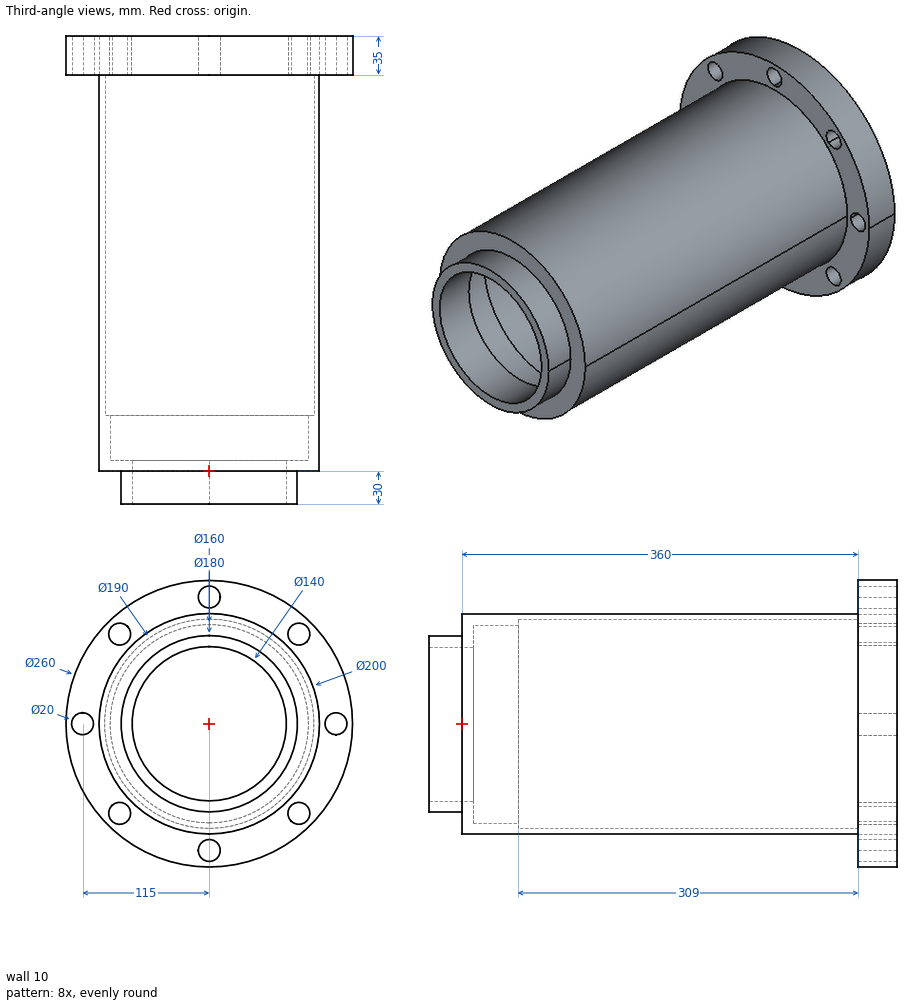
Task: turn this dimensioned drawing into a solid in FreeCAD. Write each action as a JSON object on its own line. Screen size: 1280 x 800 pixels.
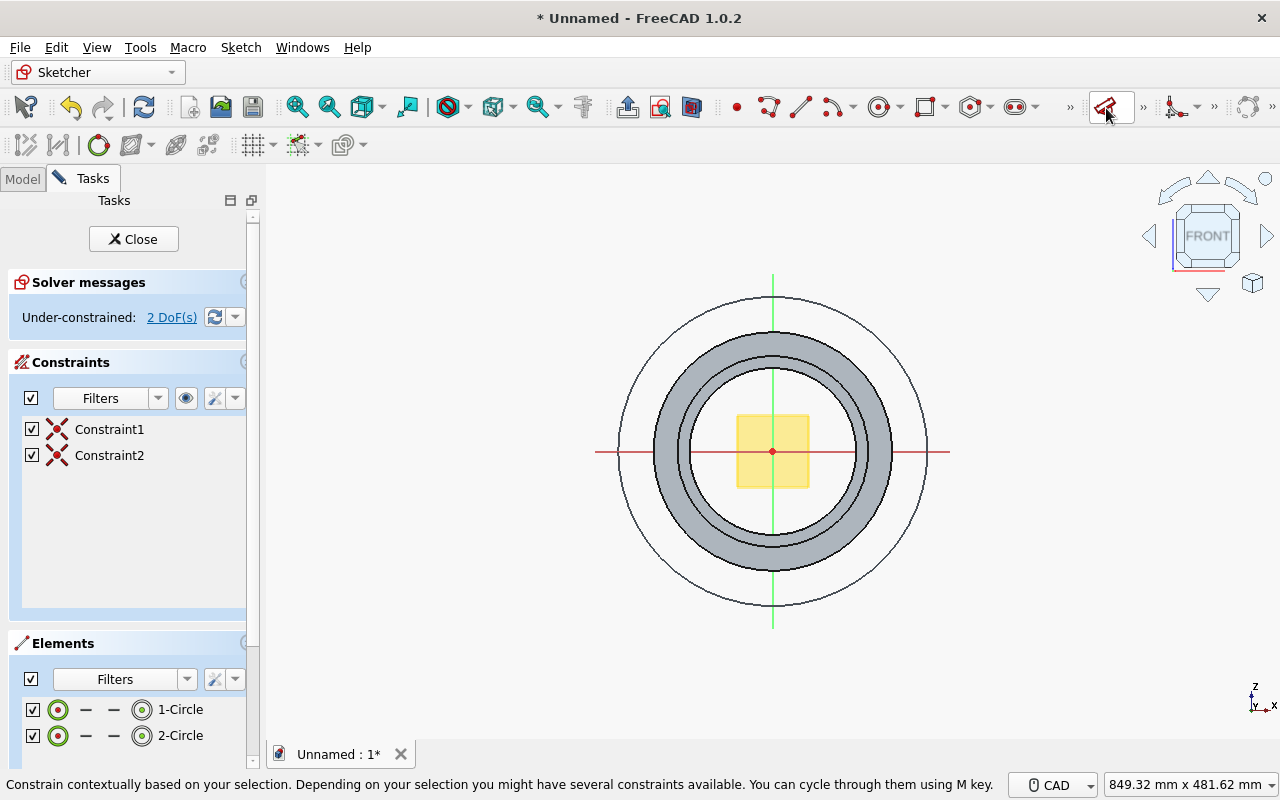
{"action": "left_click", "coordinate": [882, 342]}
{"action": "left_click", "coordinate": [905, 319]}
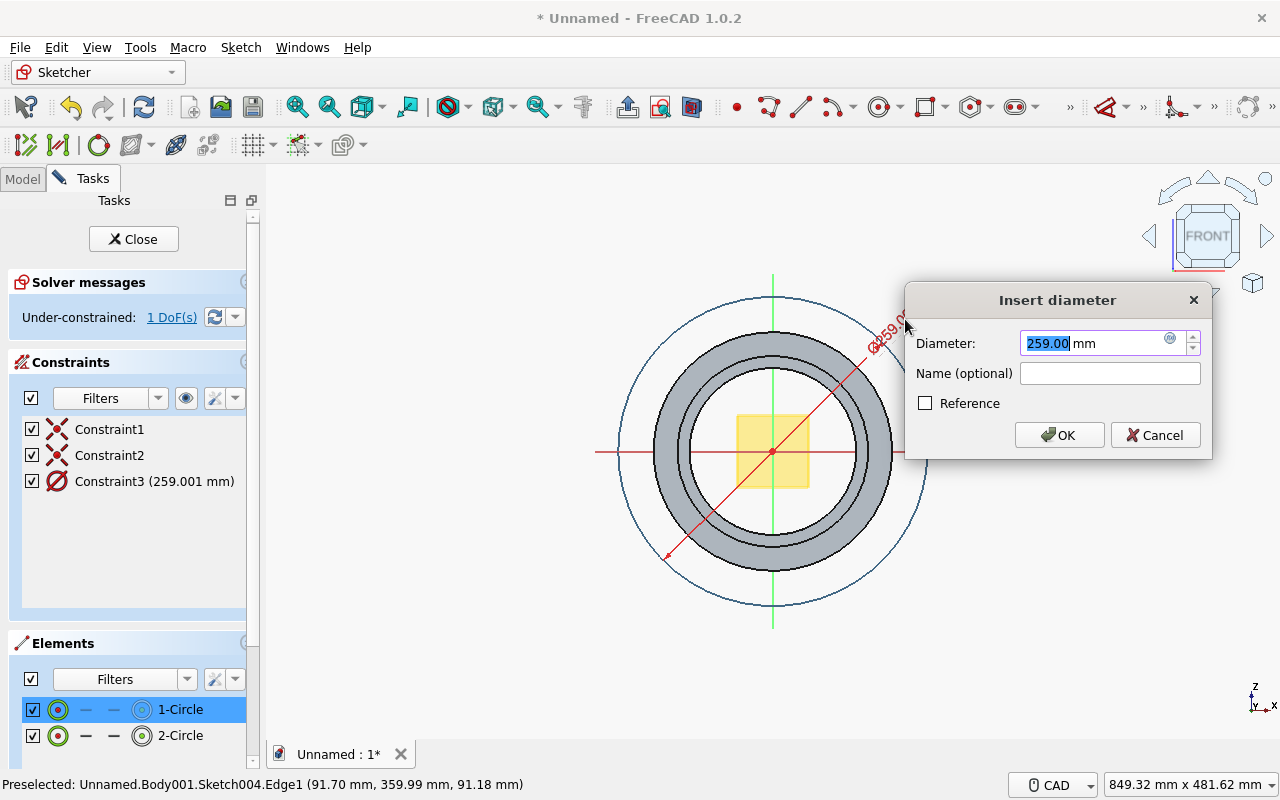
{"action": "type", "text": "260"}
{"action": "key", "text": "Return"}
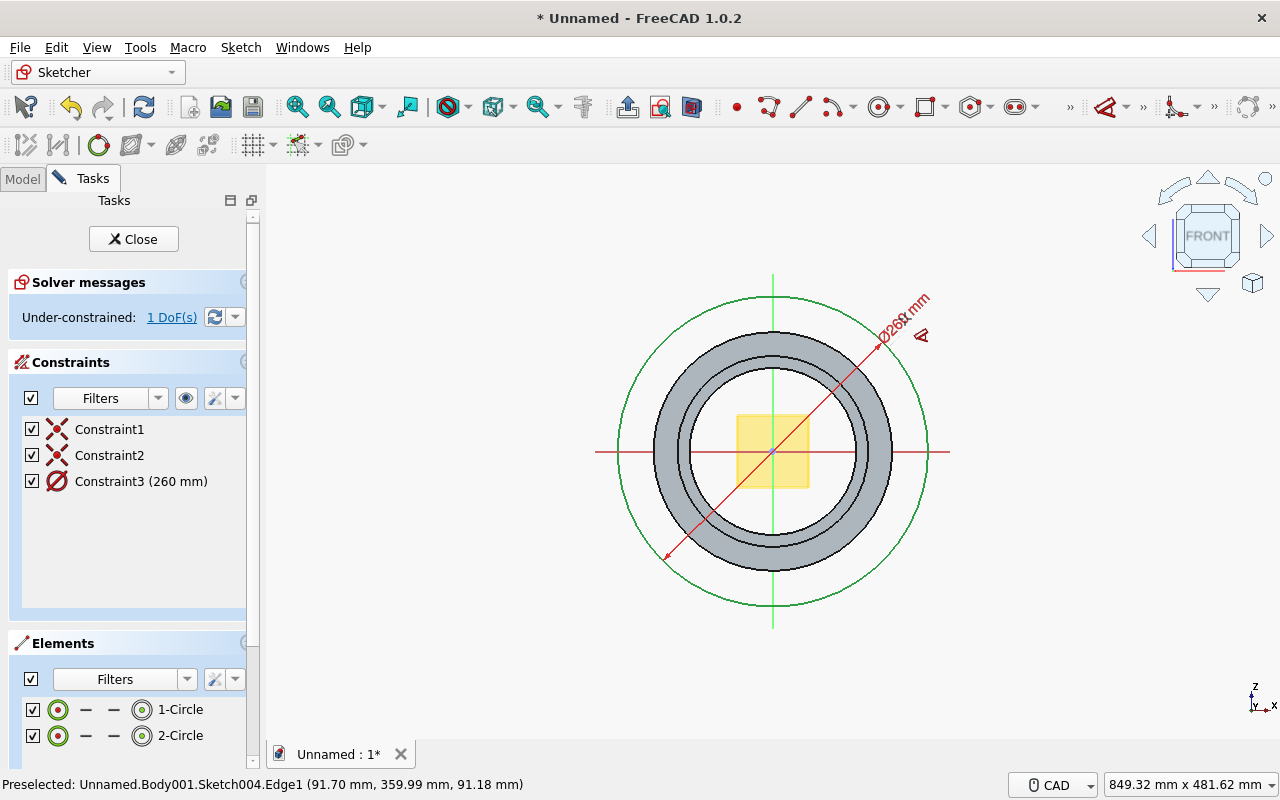
{"action": "left_click", "coordinate": [856, 367]}
{"action": "left_click", "coordinate": [939, 401]}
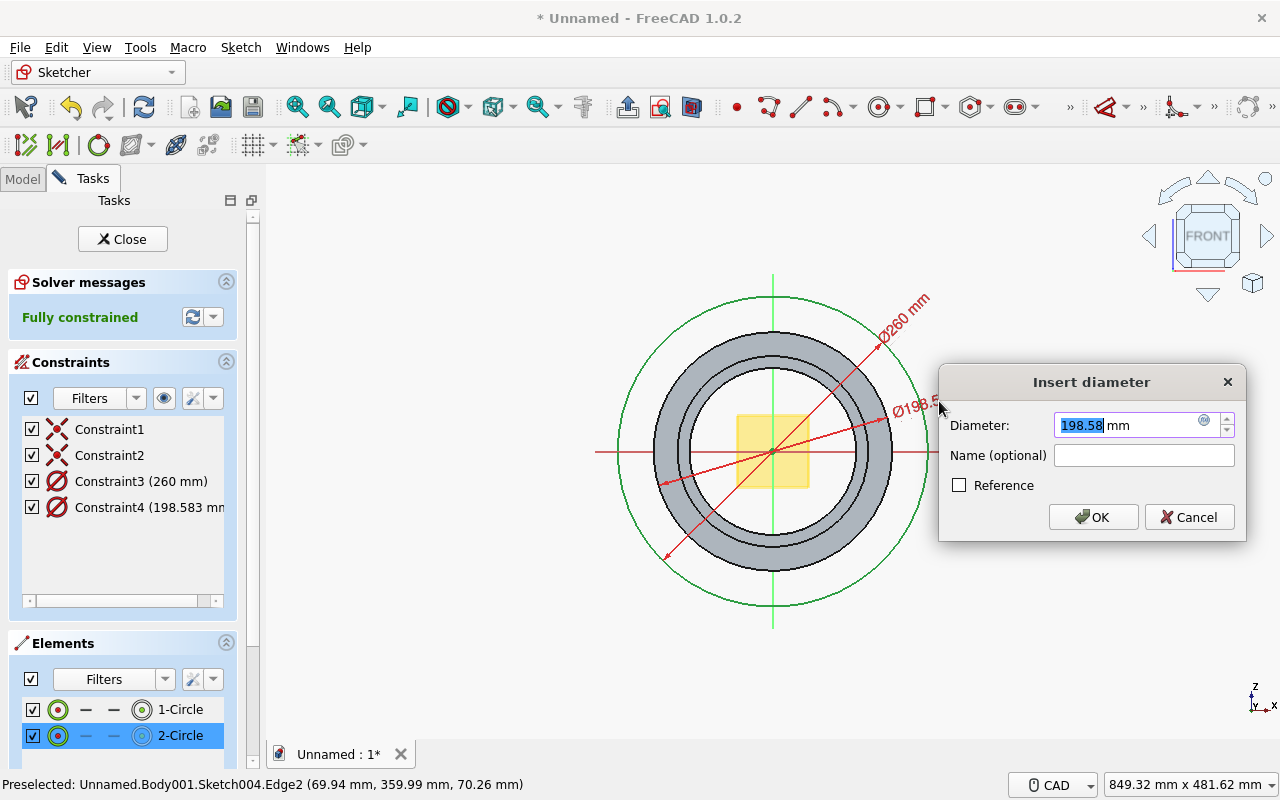
{"action": "type", "text": "200"}
{"action": "key", "text": "Return"}
{"action": "key", "text": "Escape"}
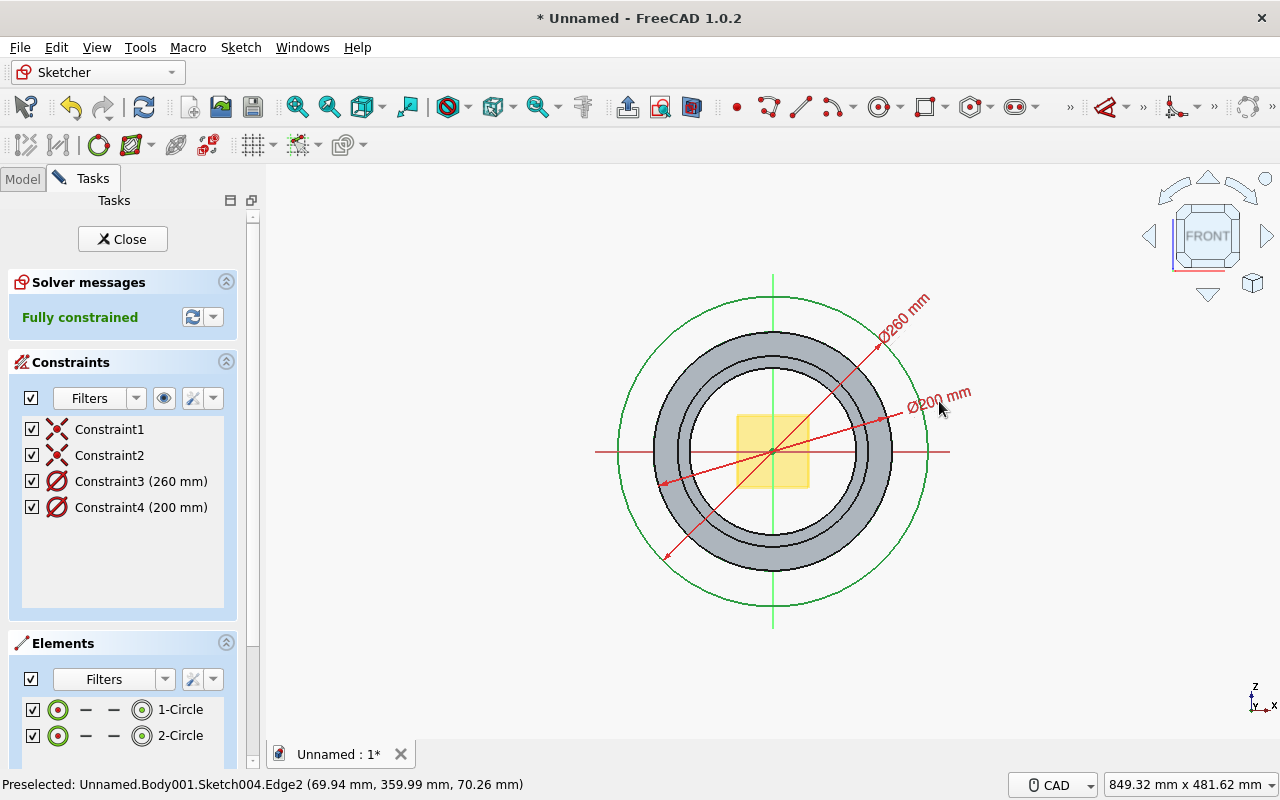
{"action": "left_click", "coordinate": [123, 239]}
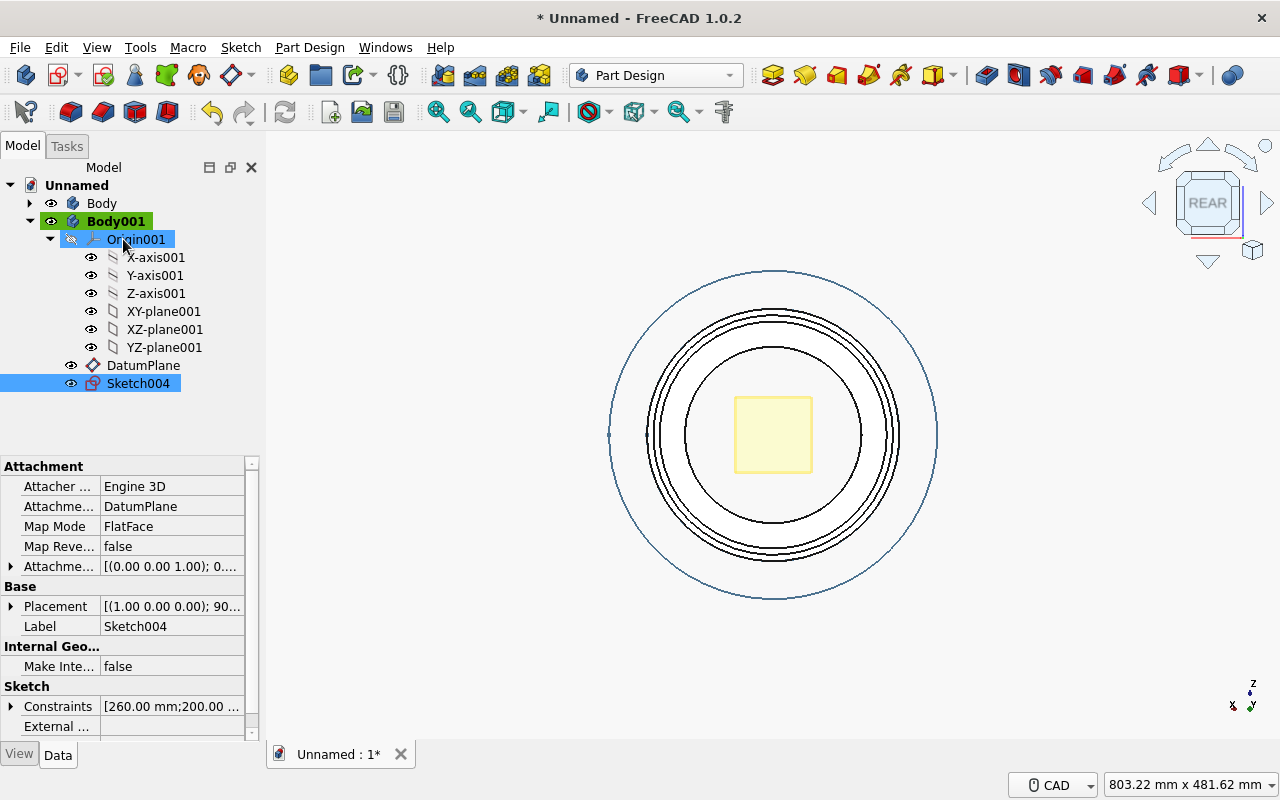
{"action": "left_click", "coordinate": [774, 76]}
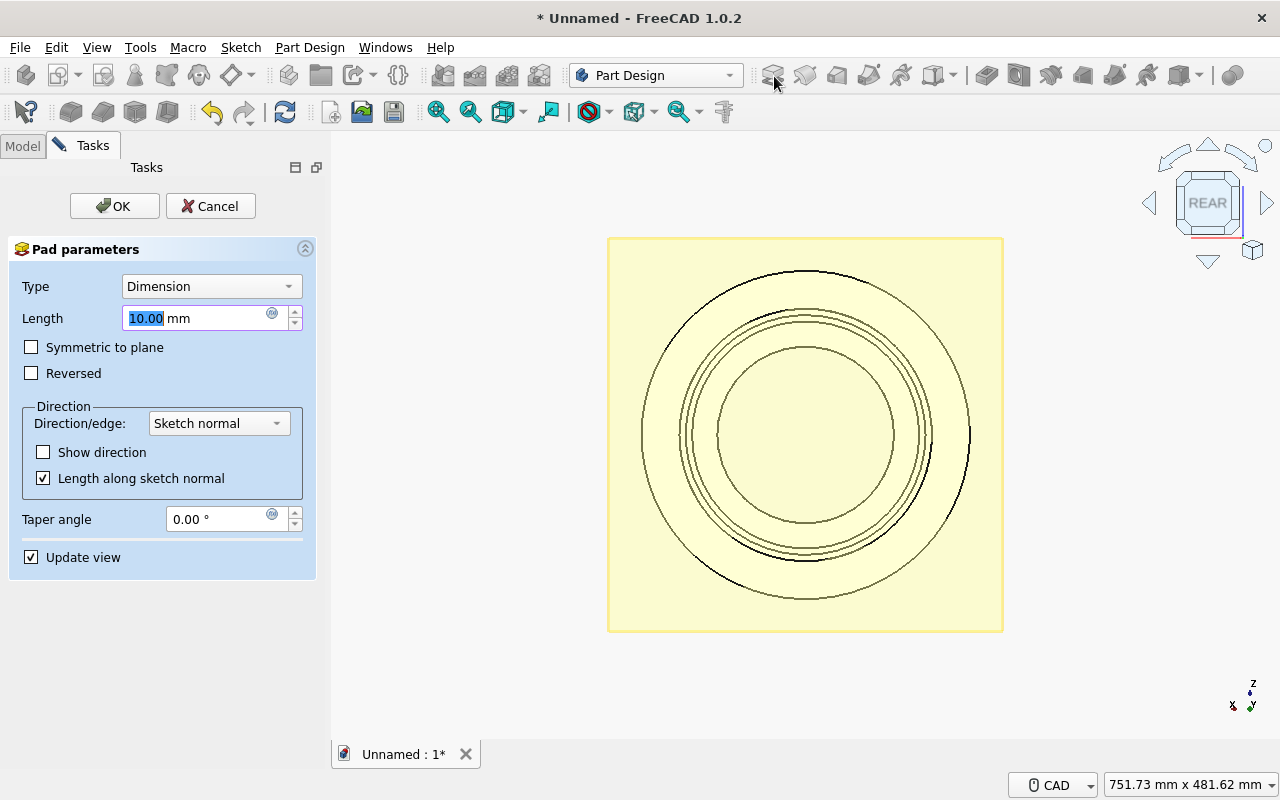
{"action": "type", "text": "35"}
{"action": "key", "text": "Tab"}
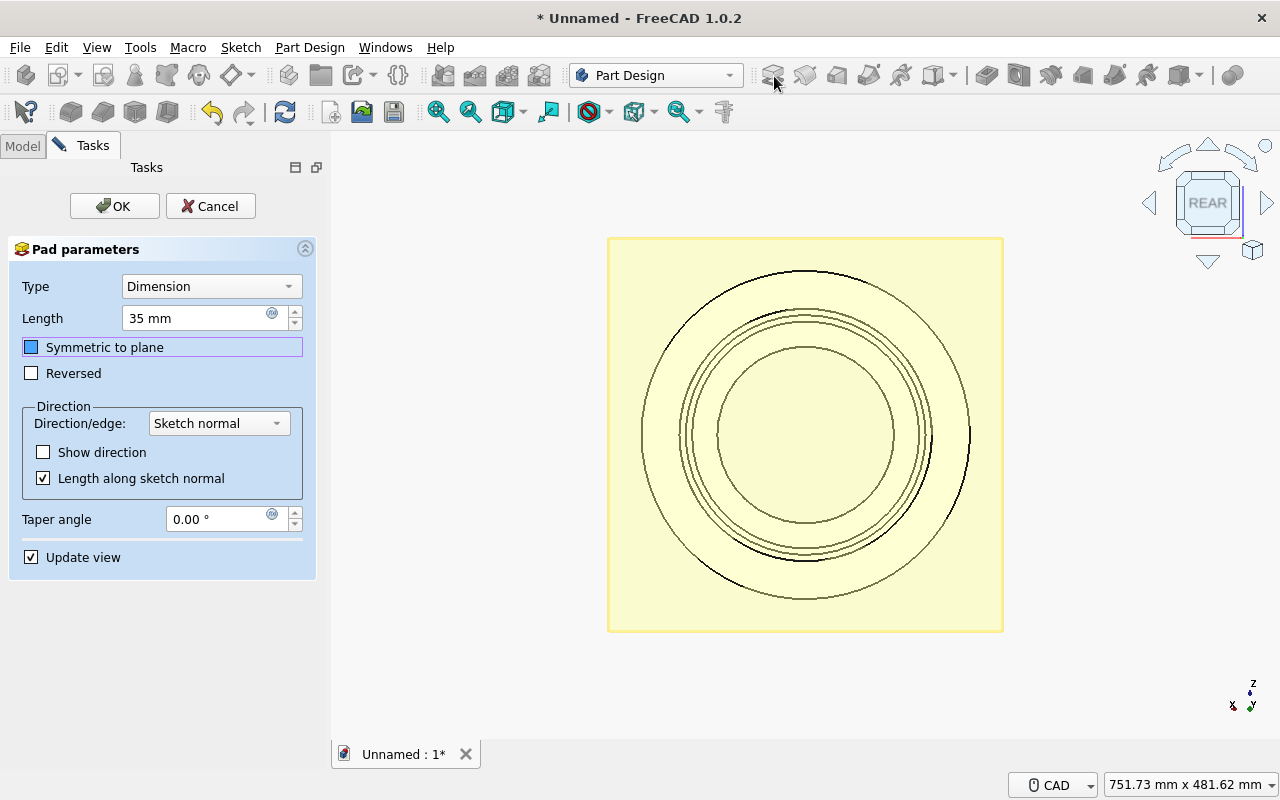
{"action": "left_click", "coordinate": [30, 373]}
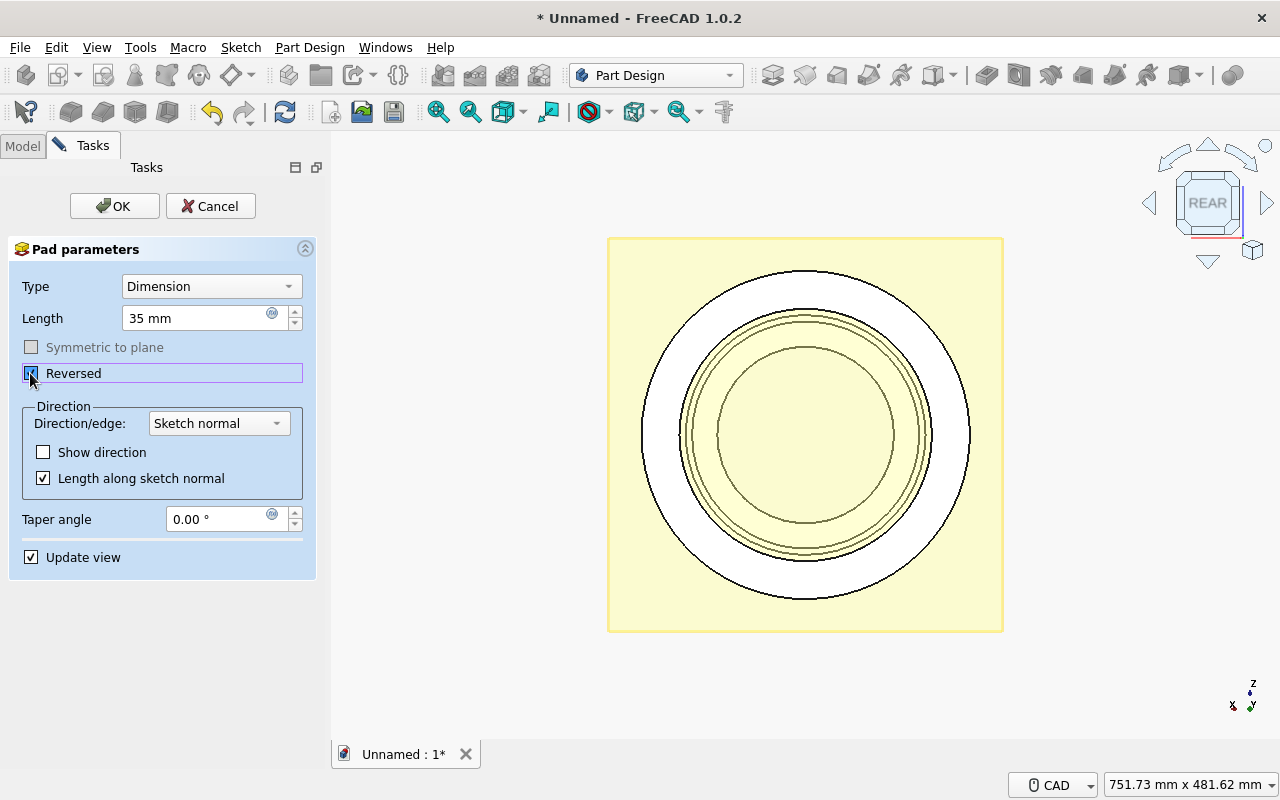
{"action": "left_click", "coordinate": [115, 206]}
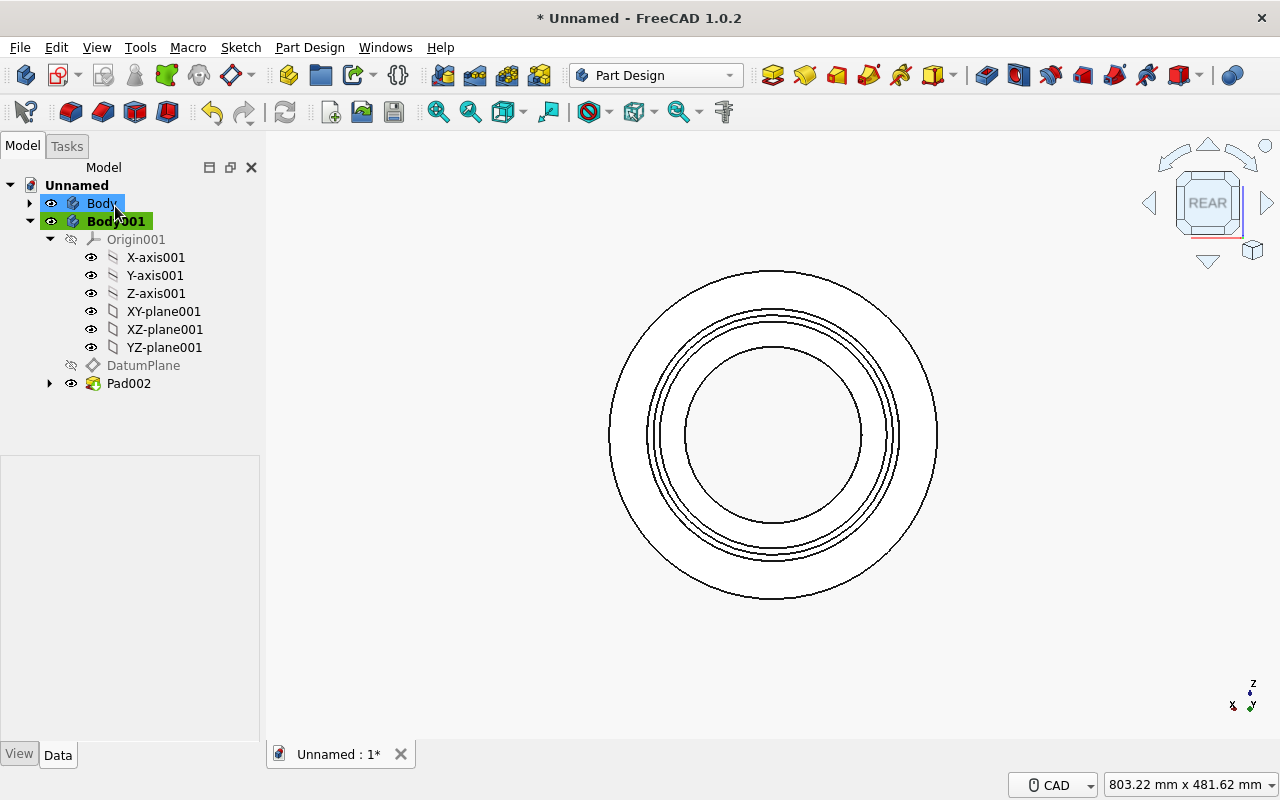
{"action": "left_click", "coordinate": [632, 481]}